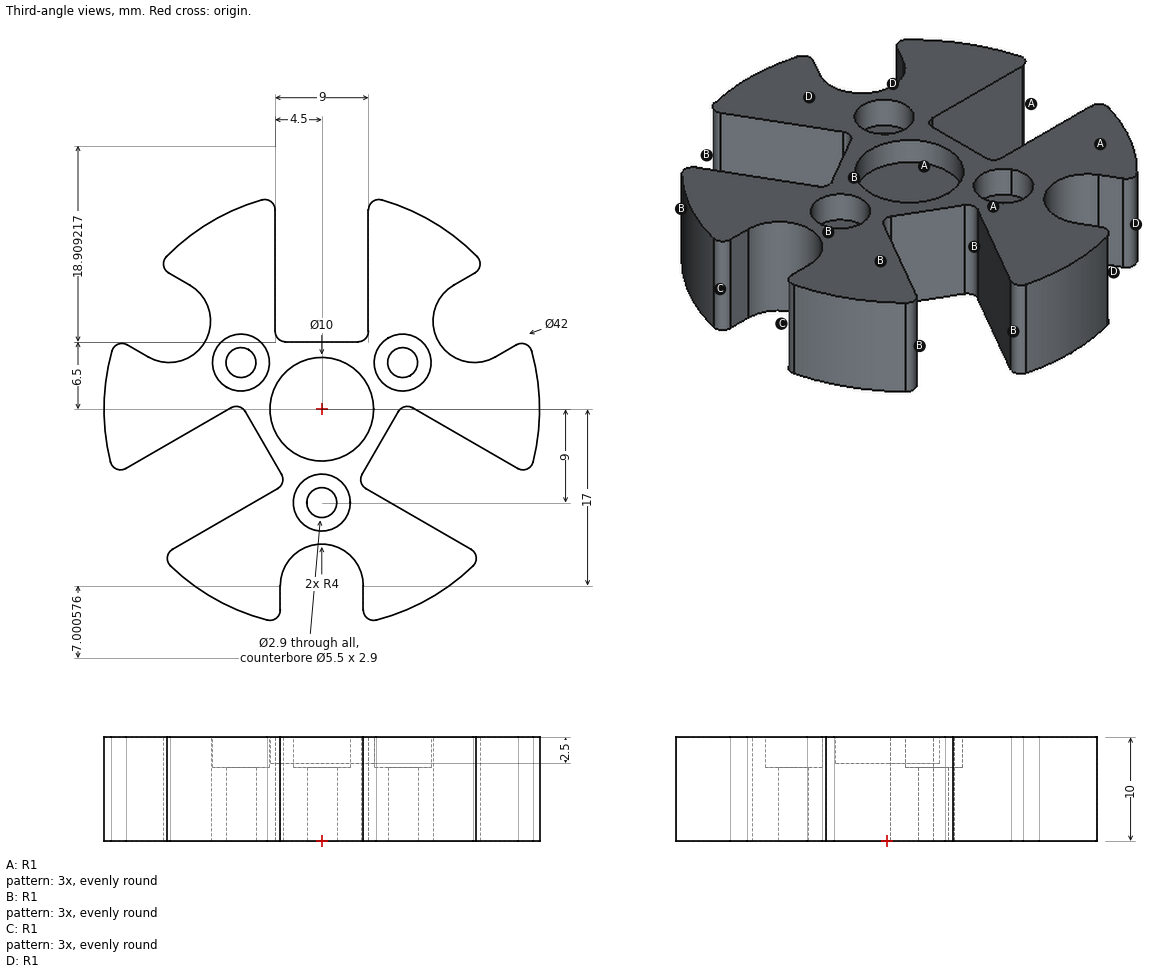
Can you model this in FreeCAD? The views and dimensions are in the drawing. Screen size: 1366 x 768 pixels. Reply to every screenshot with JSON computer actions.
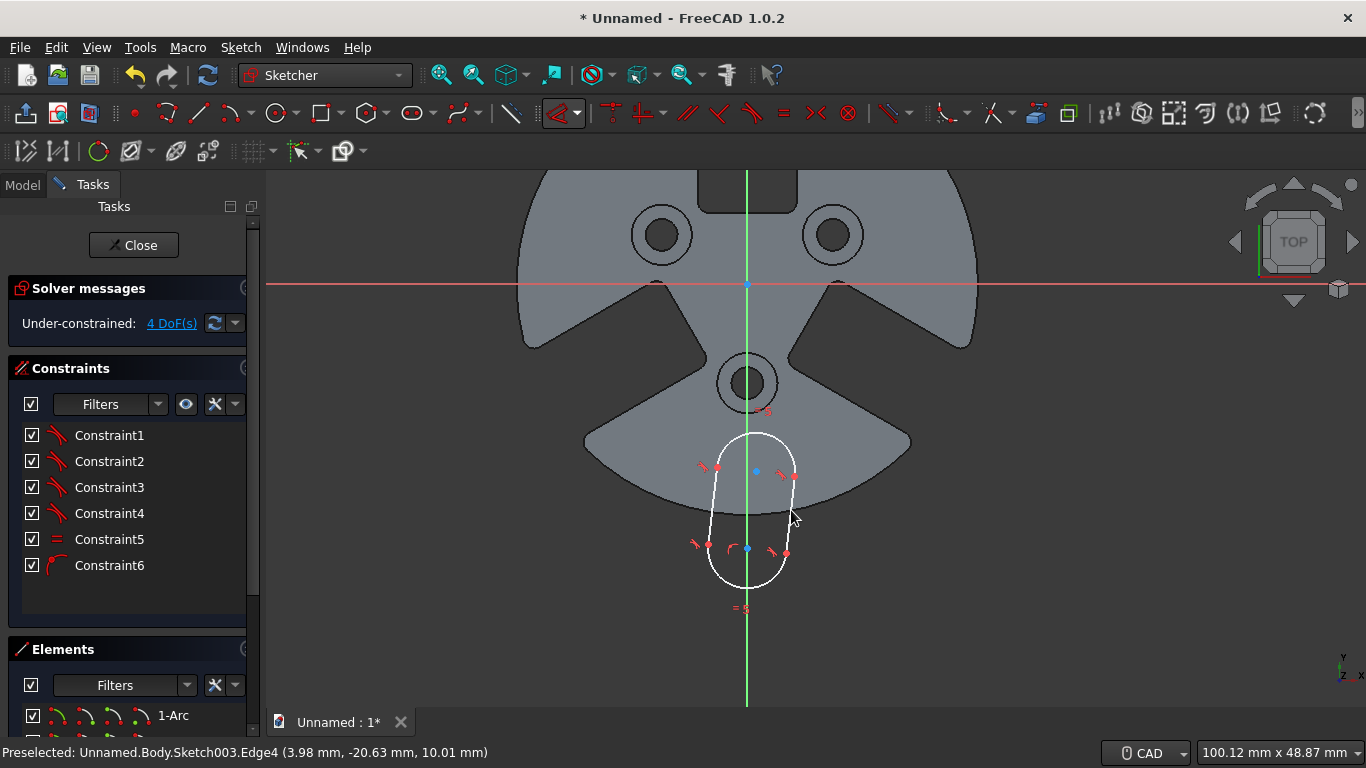
{"action": "left_click", "coordinate": [711, 522]}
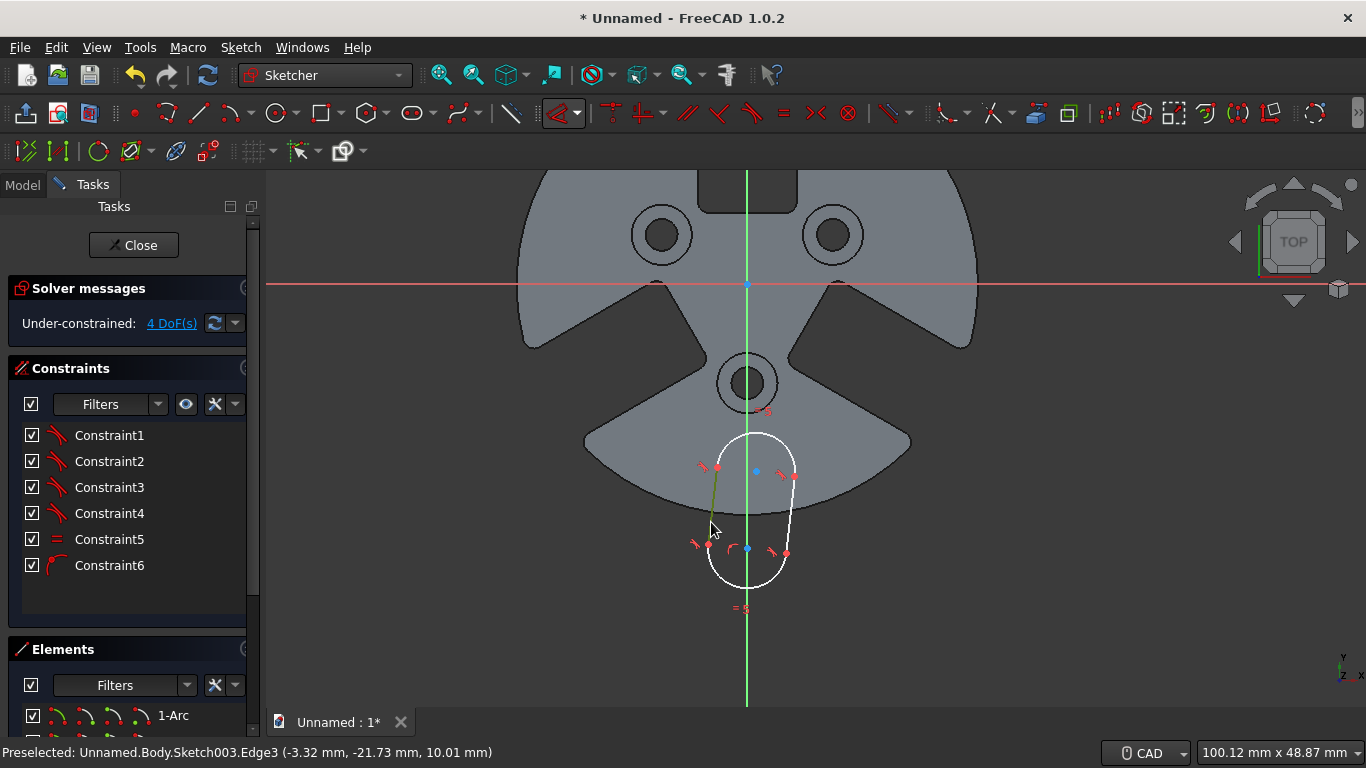
{"action": "left_click", "coordinate": [666, 114]}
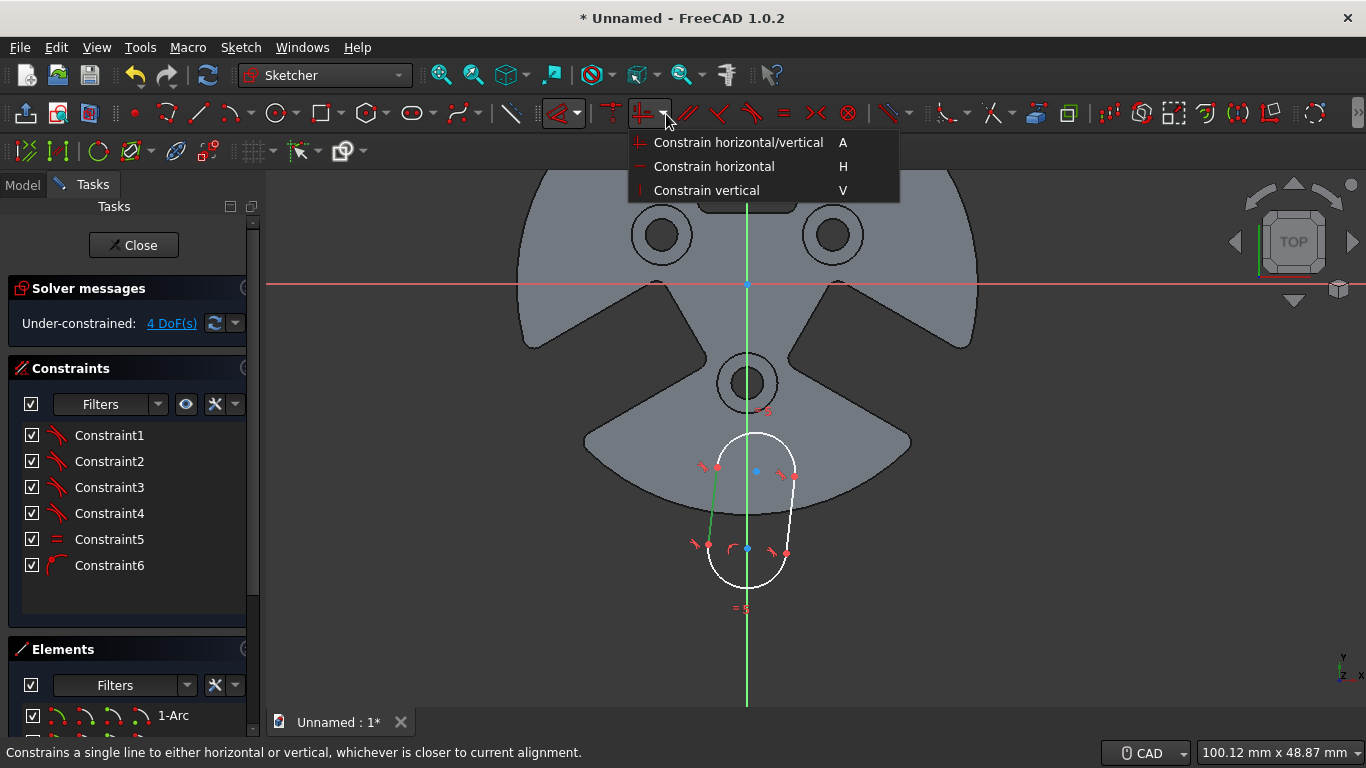
{"action": "left_click", "coordinate": [764, 190]}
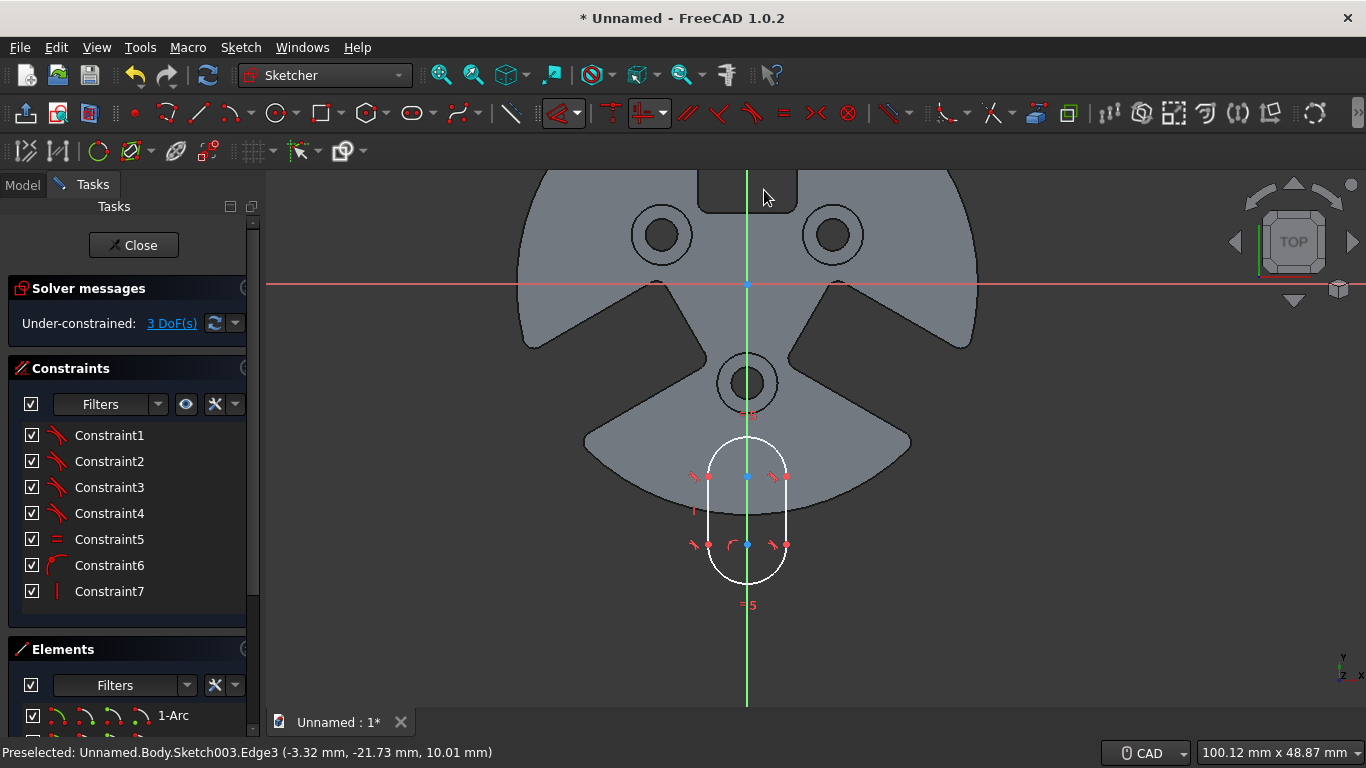
{"action": "left_click", "coordinate": [724, 576]}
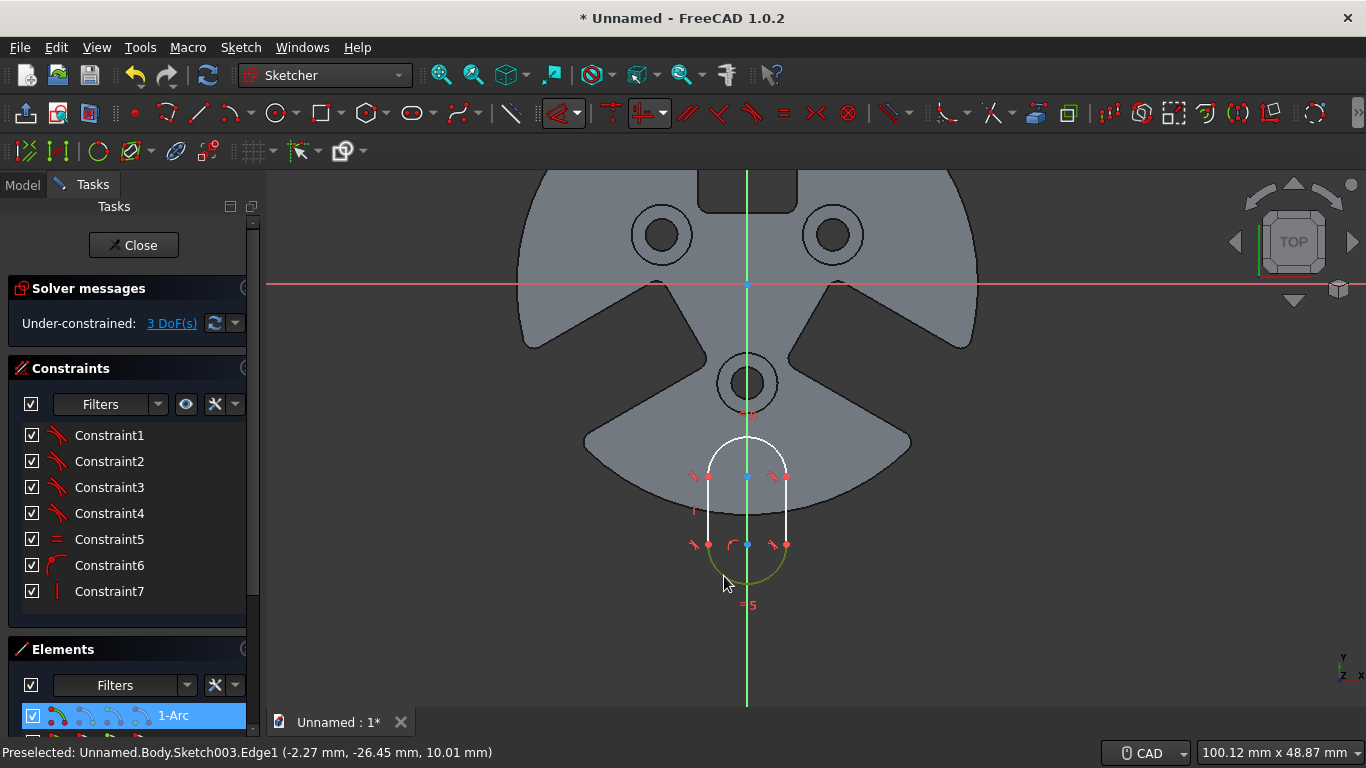
{"action": "key", "text": "k r"}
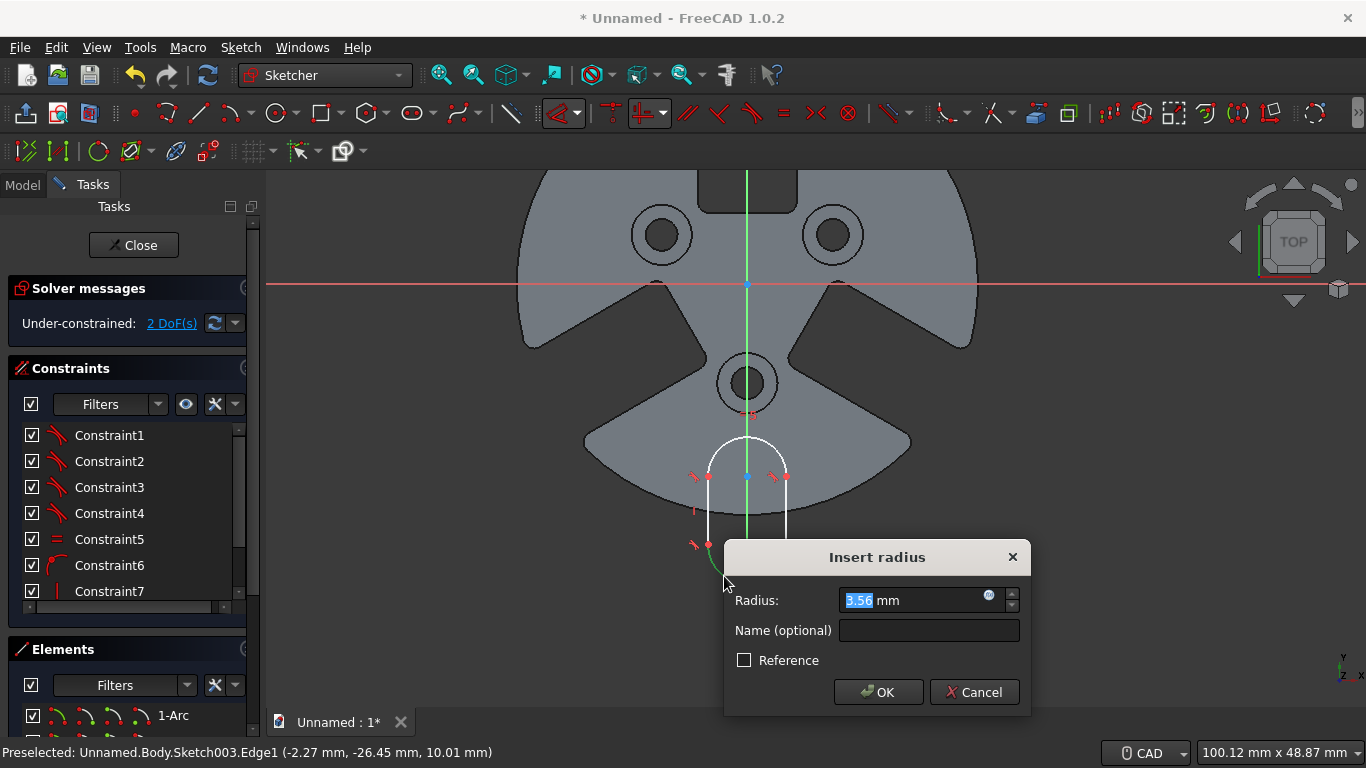
{"action": "type", "text": "4"}
{"action": "key", "text": "Return"}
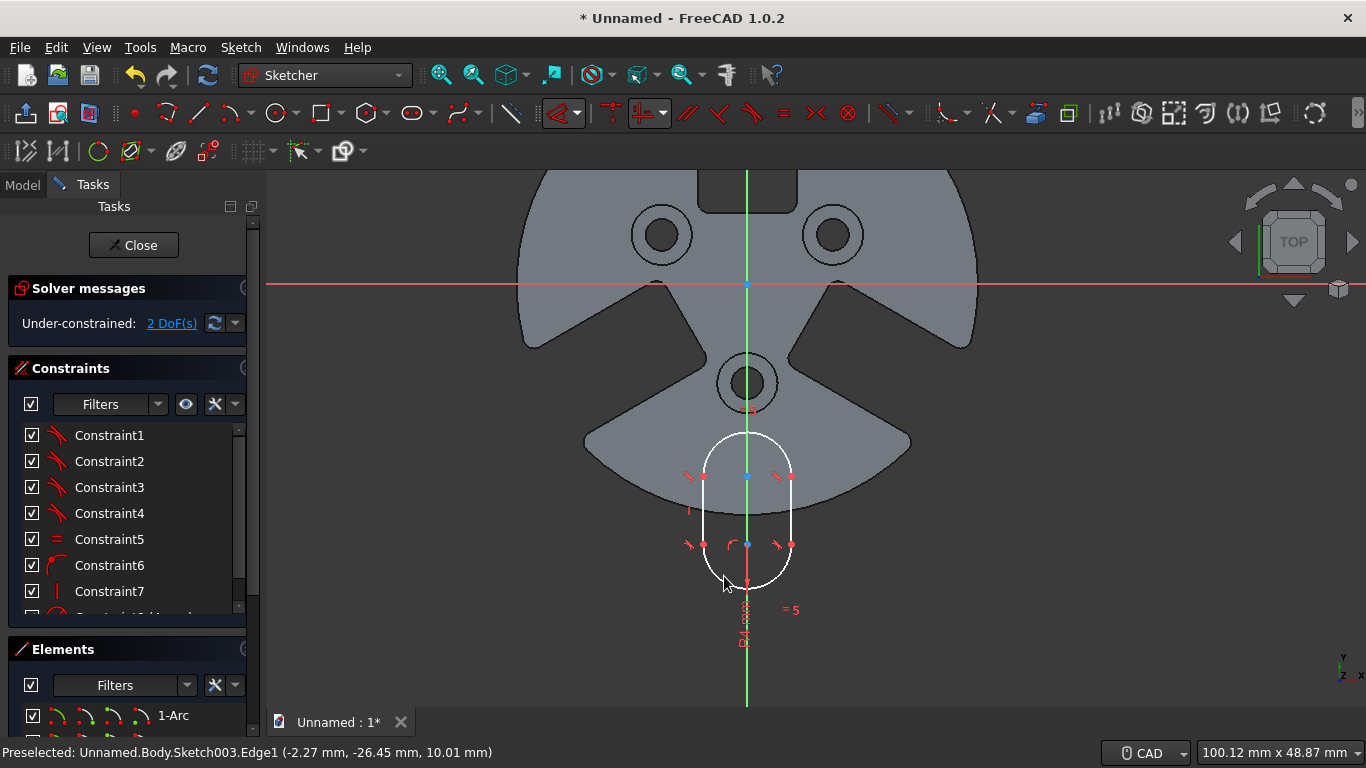
{"action": "left_click", "coordinate": [791, 476]}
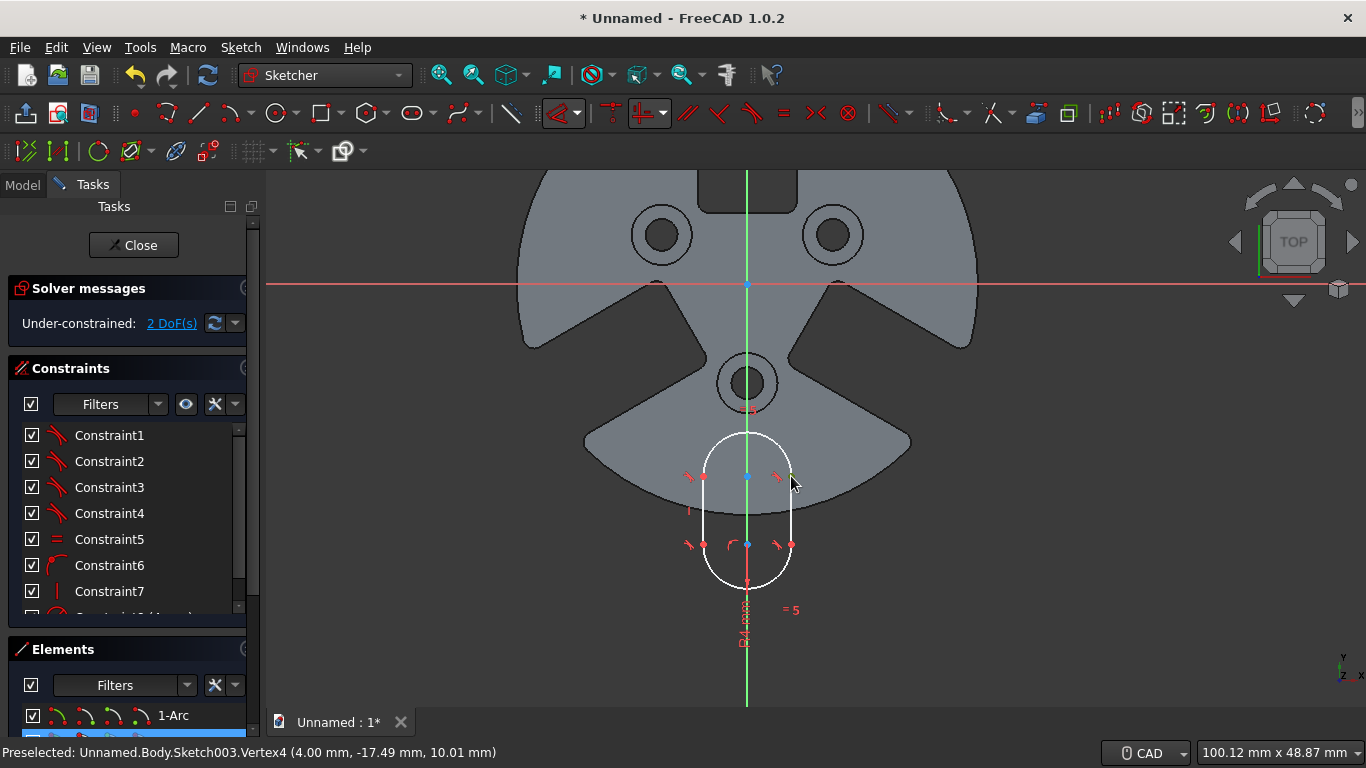
{"action": "key", "text": "i"}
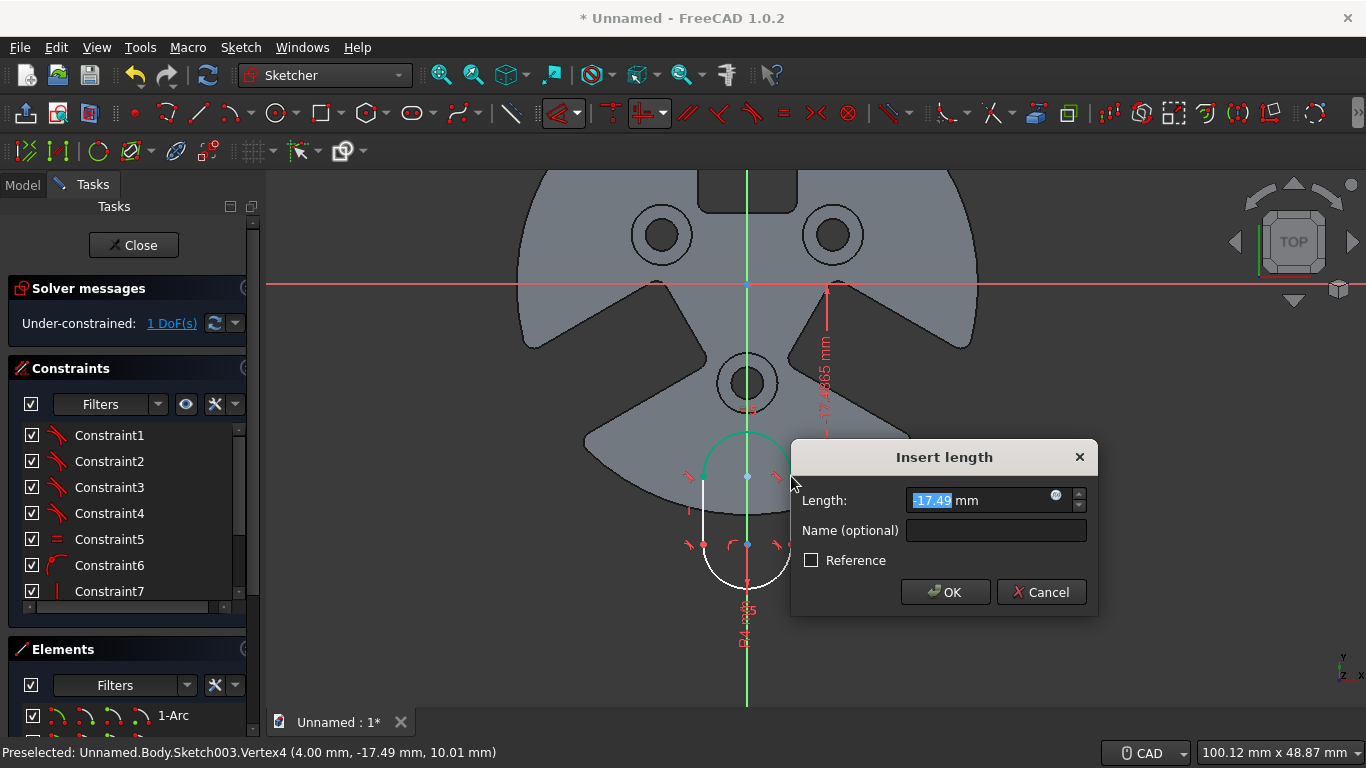
{"action": "type", "text": "-17"}
{"action": "key", "text": "Return"}